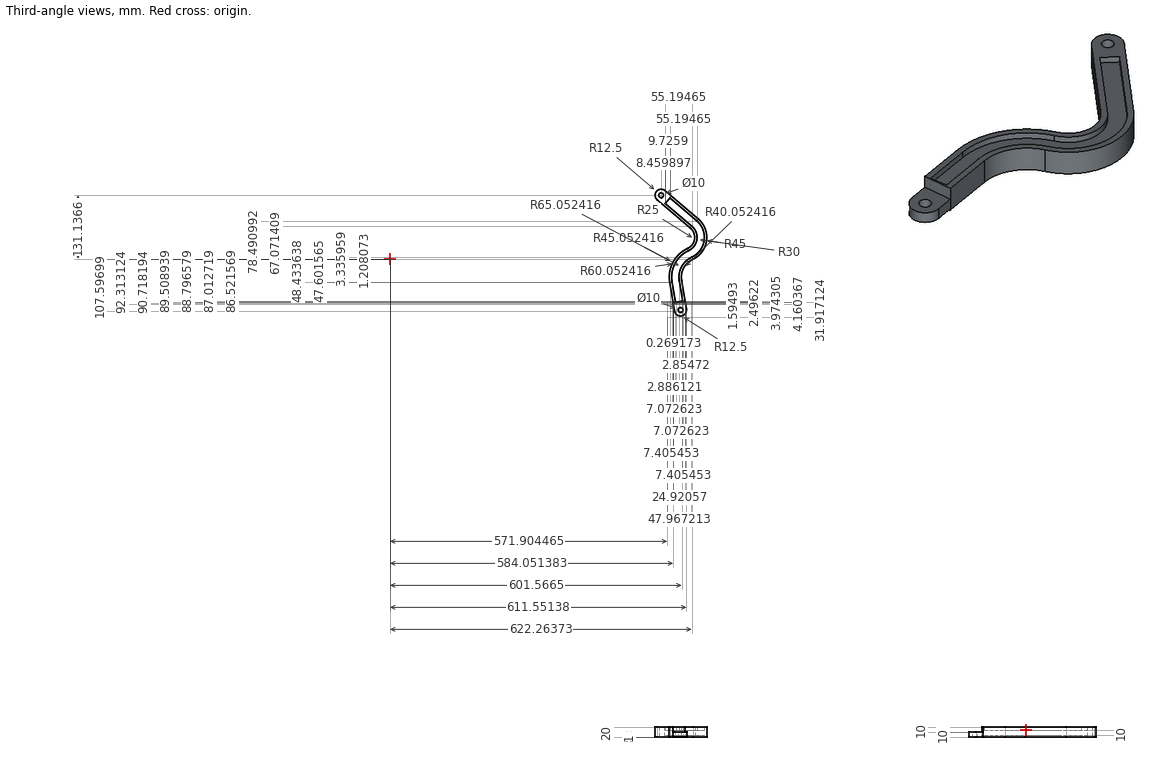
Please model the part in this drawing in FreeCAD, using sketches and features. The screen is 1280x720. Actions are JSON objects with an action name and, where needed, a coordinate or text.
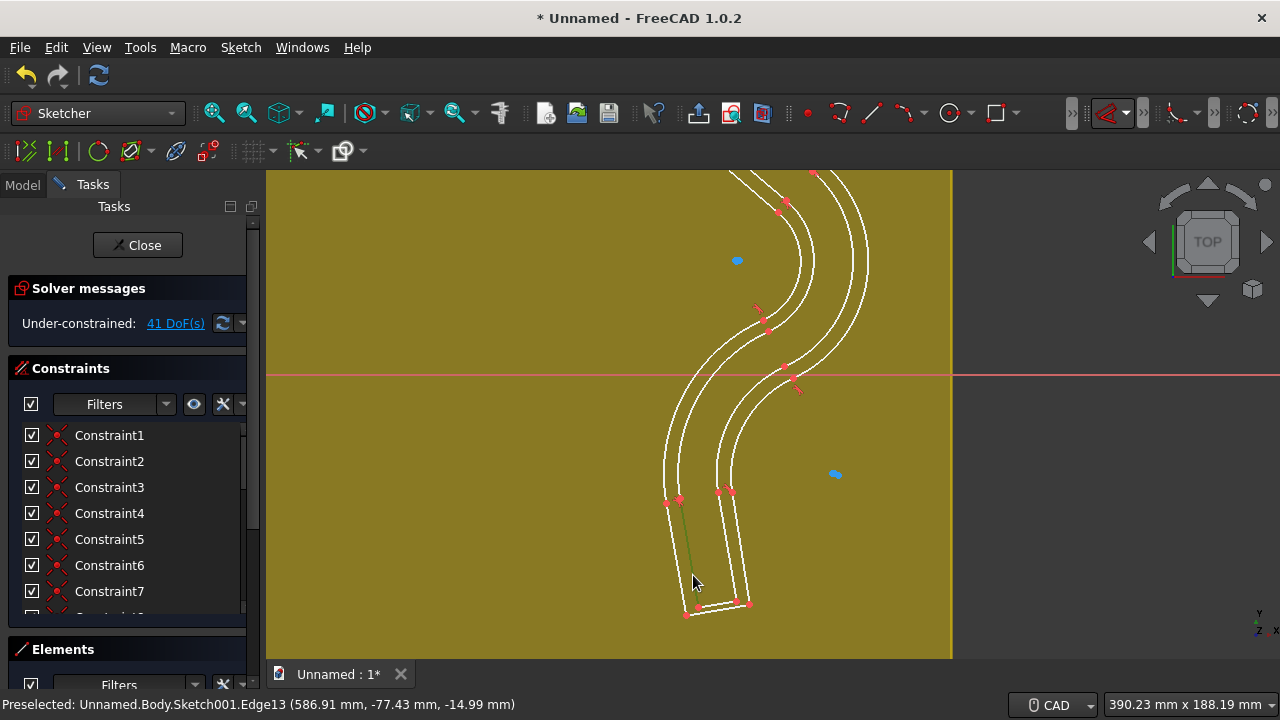
{"action": "left_click", "coordinate": [682, 438]}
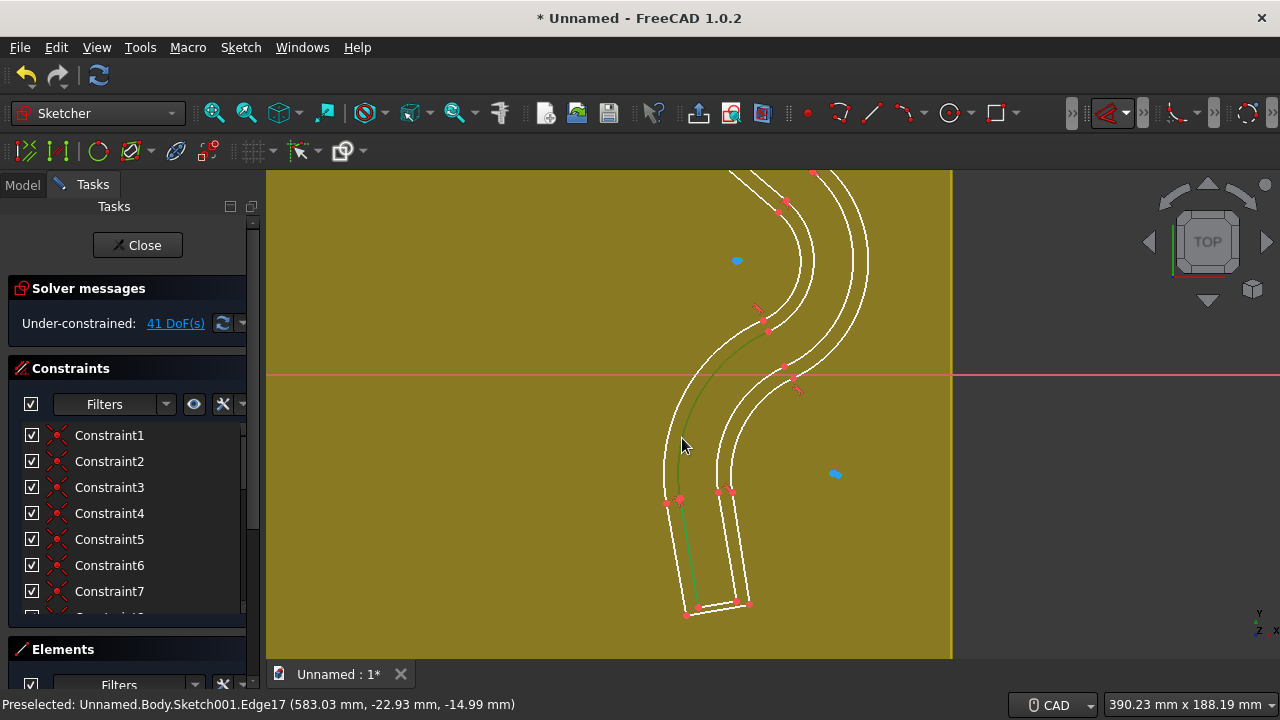
{"action": "key", "text": "t"}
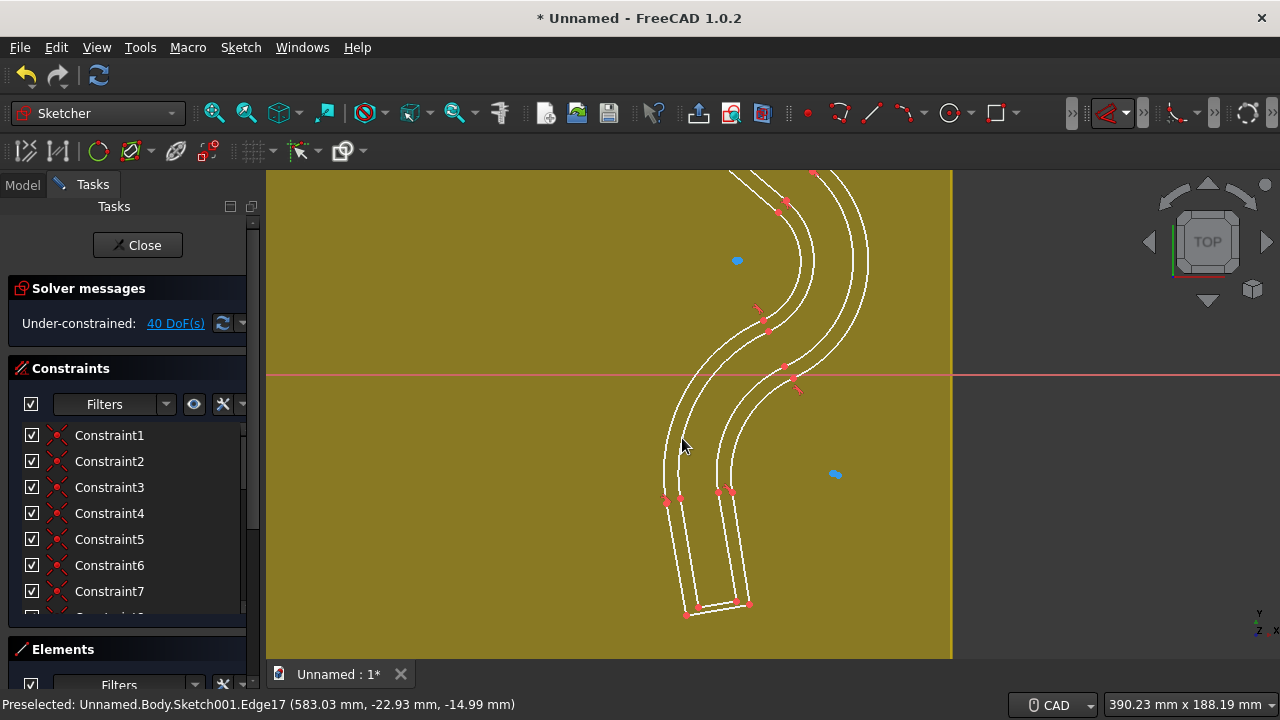
{"action": "scroll", "coordinate": [672, 539], "scroll_direction": "down", "scroll_amount": 3}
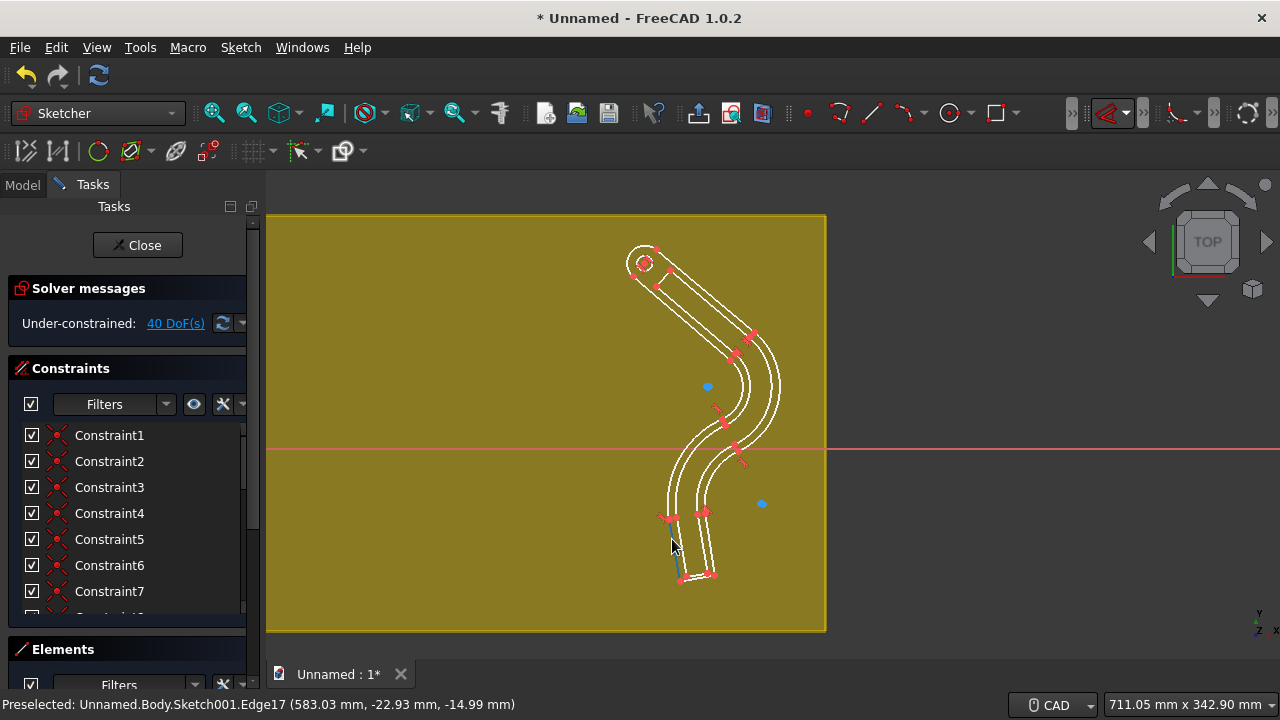
{"action": "scroll", "coordinate": [711, 334], "scroll_direction": "up", "scroll_amount": 3}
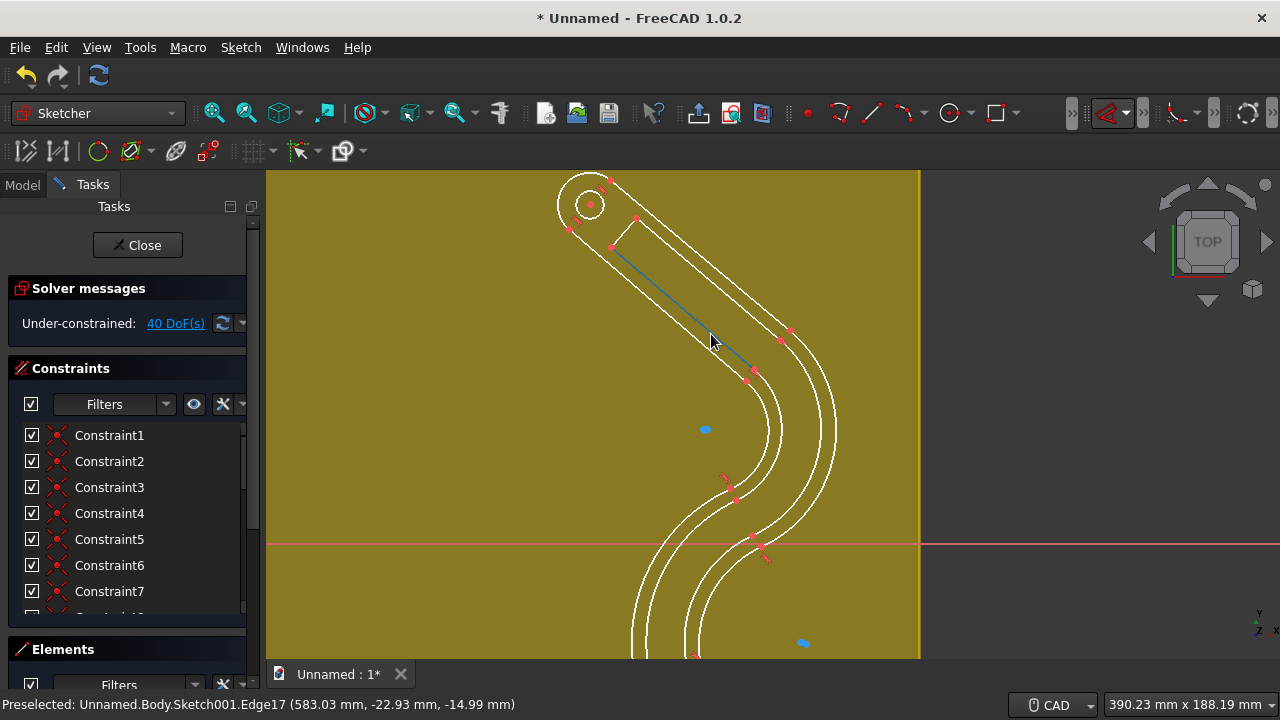
{"action": "left_click", "coordinate": [712, 333]}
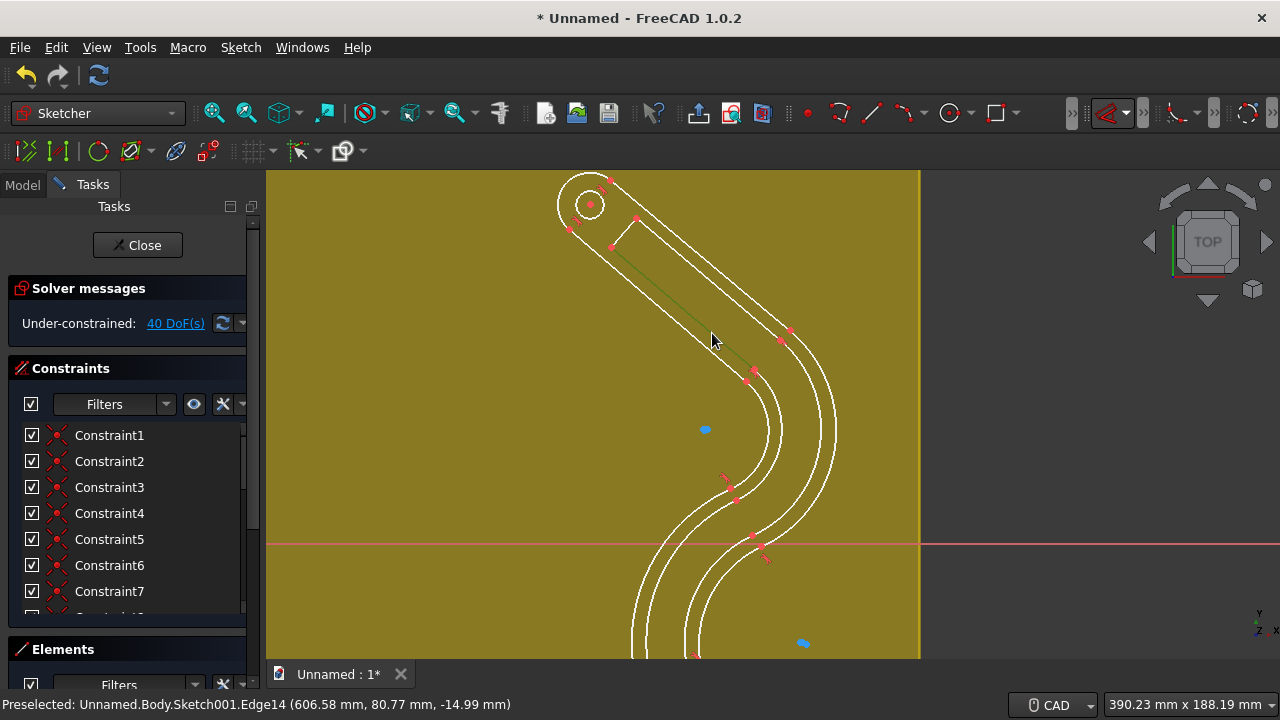
{"action": "left_click", "coordinate": [771, 469]}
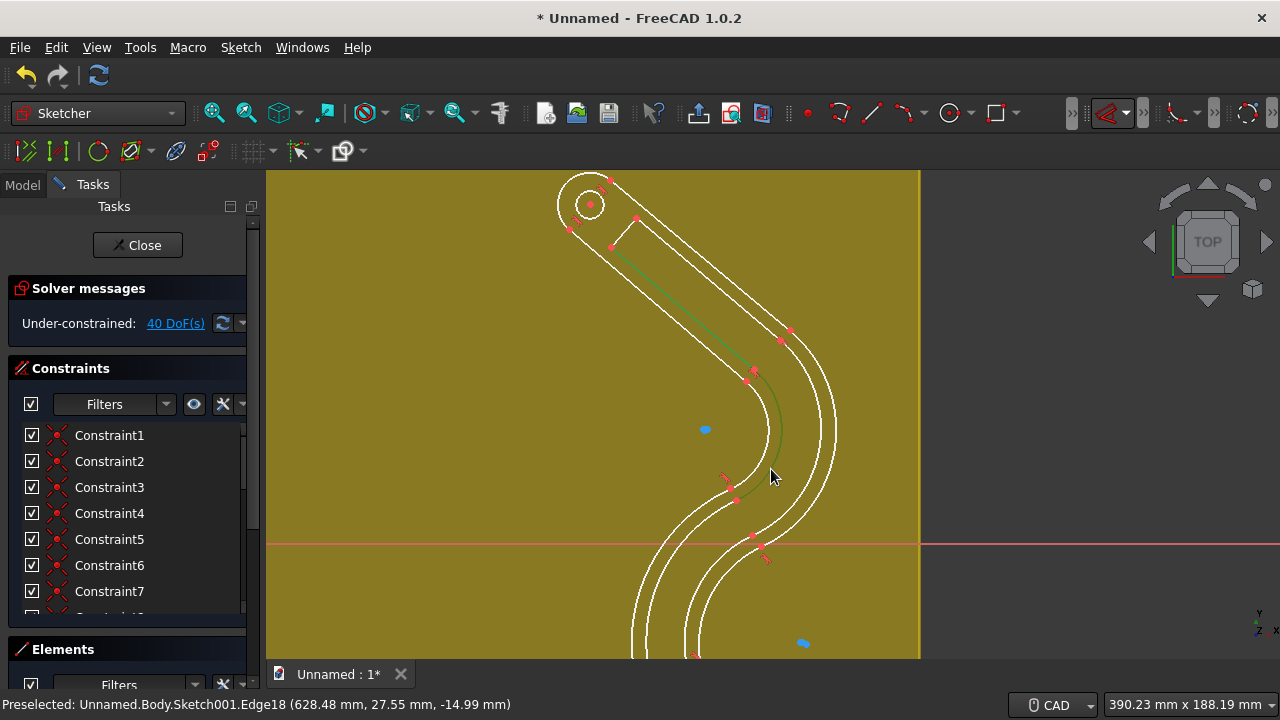
{"action": "key", "text": "t"}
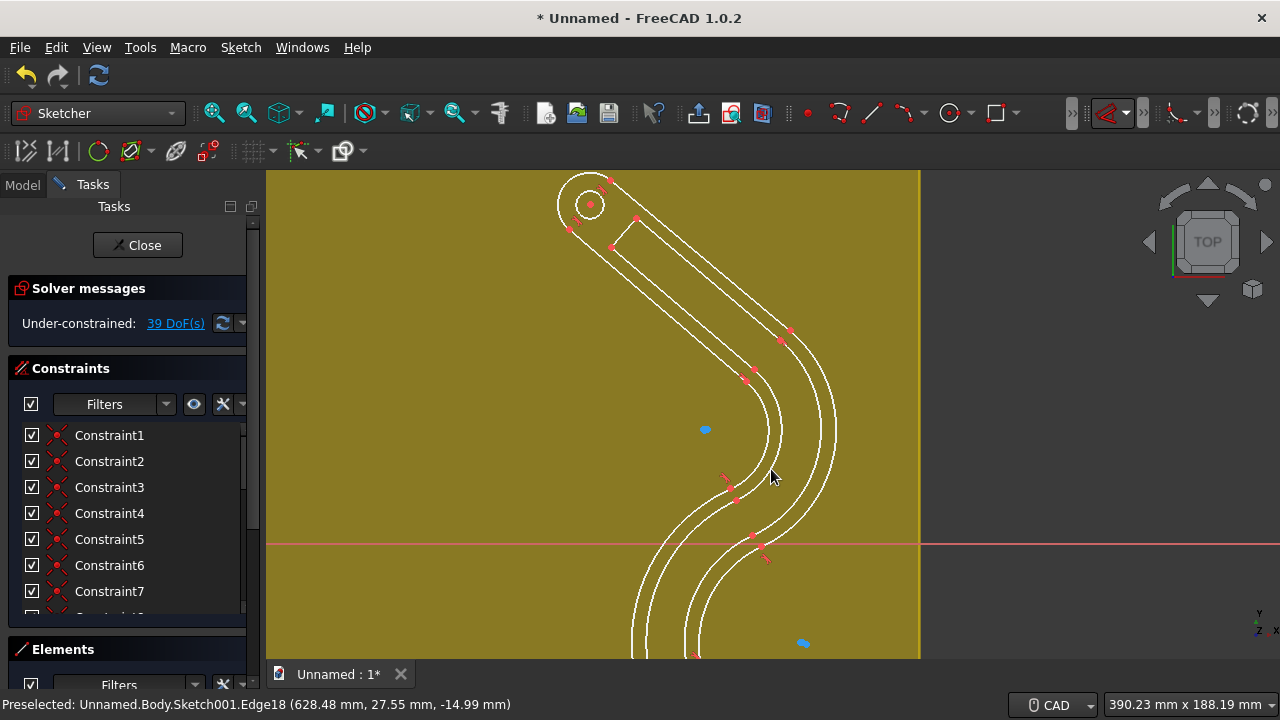
{"action": "left_click", "coordinate": [680, 255]}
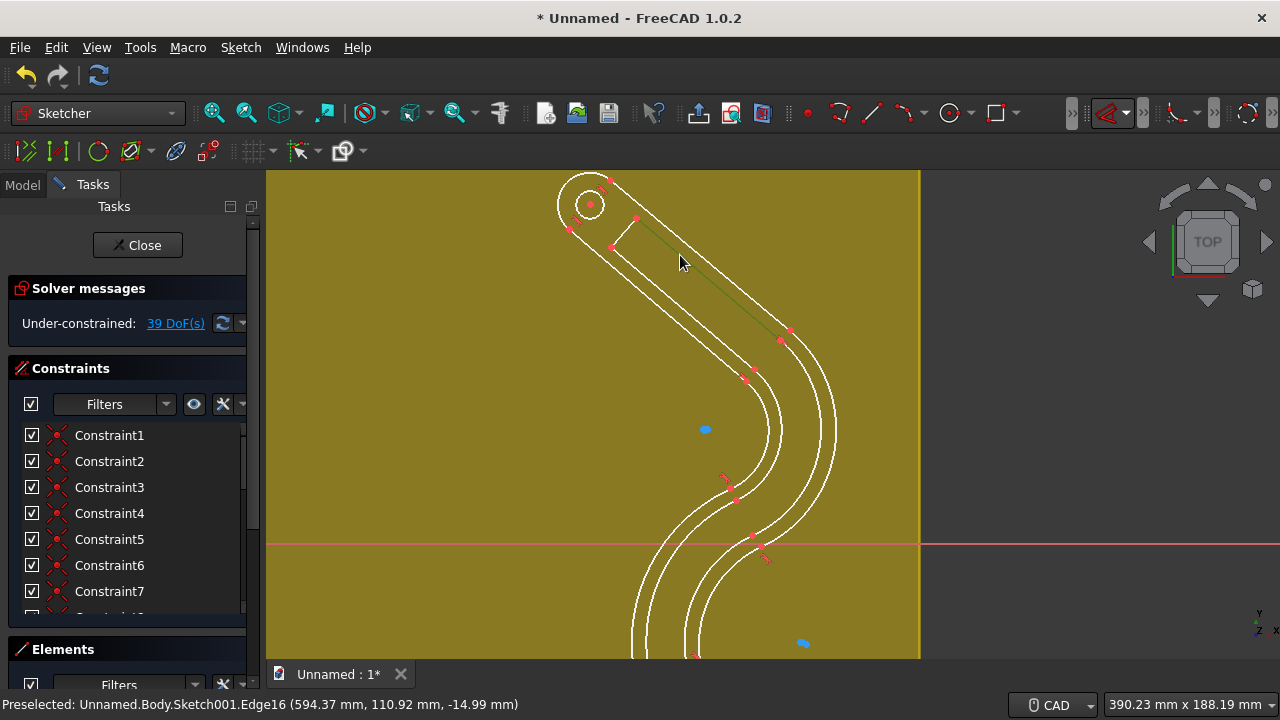
{"action": "left_click", "coordinate": [804, 489]}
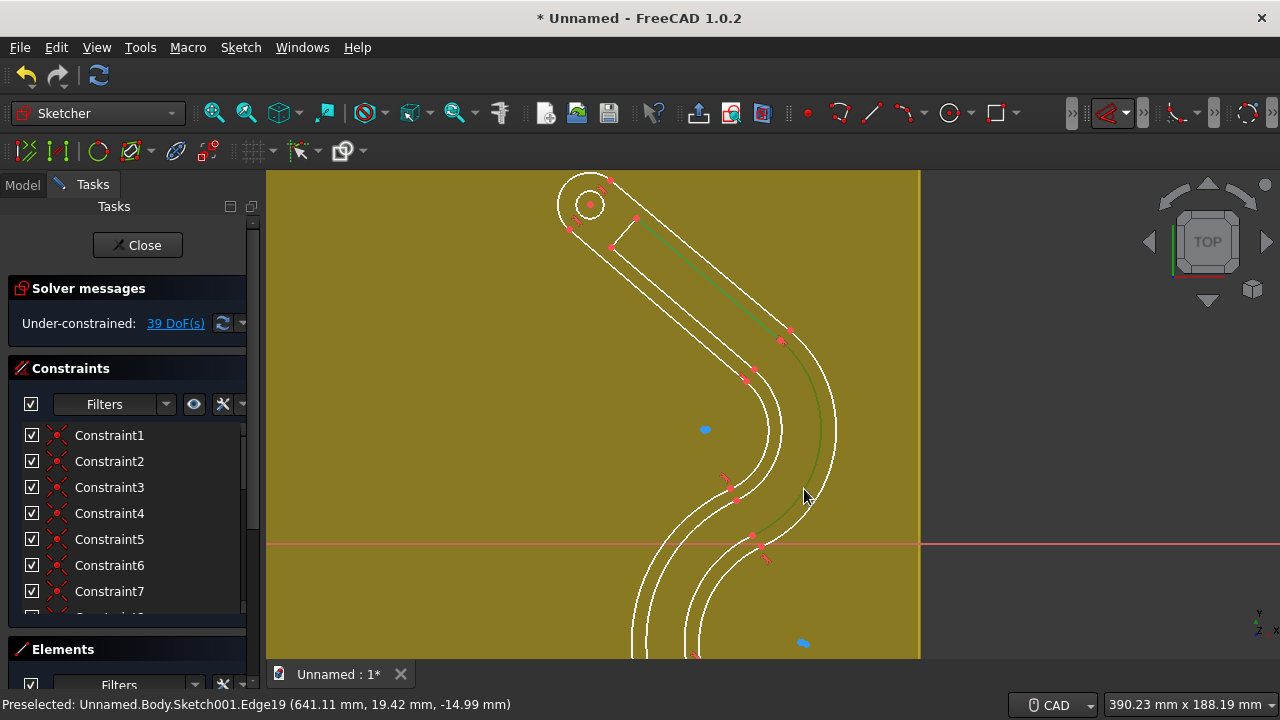
{"action": "key", "text": "t"}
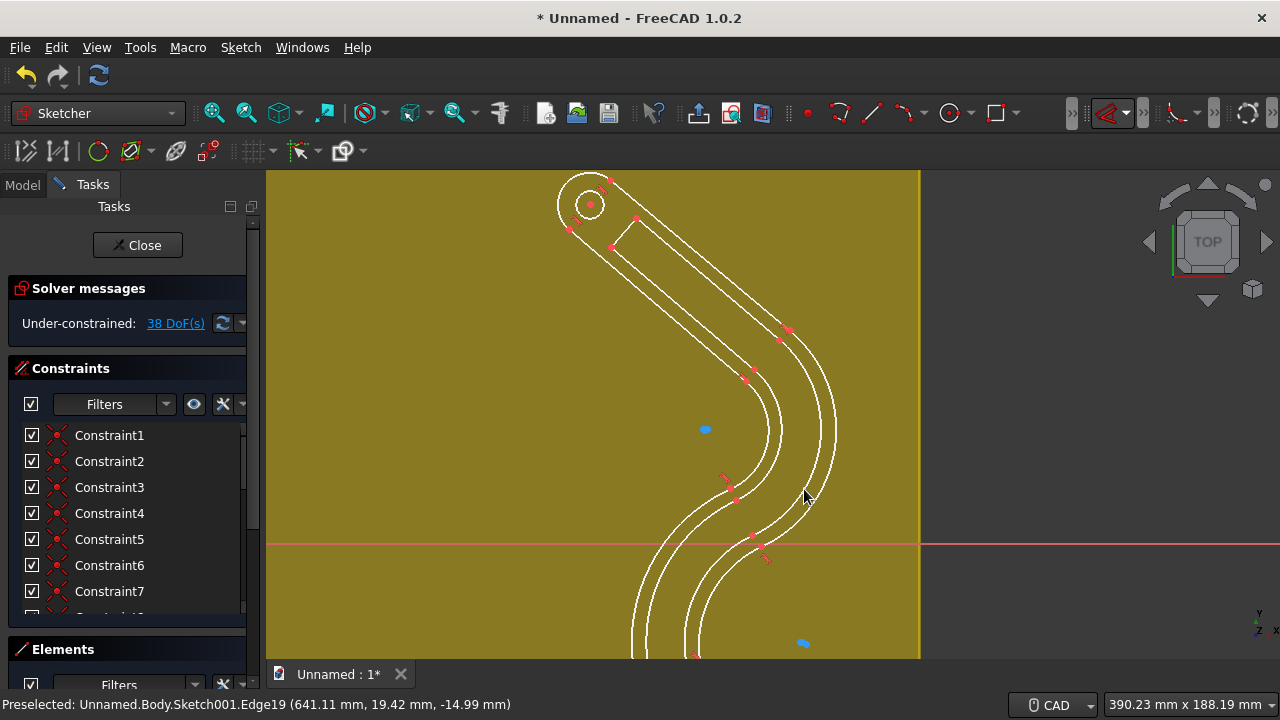
{"action": "left_click", "coordinate": [650, 607]}